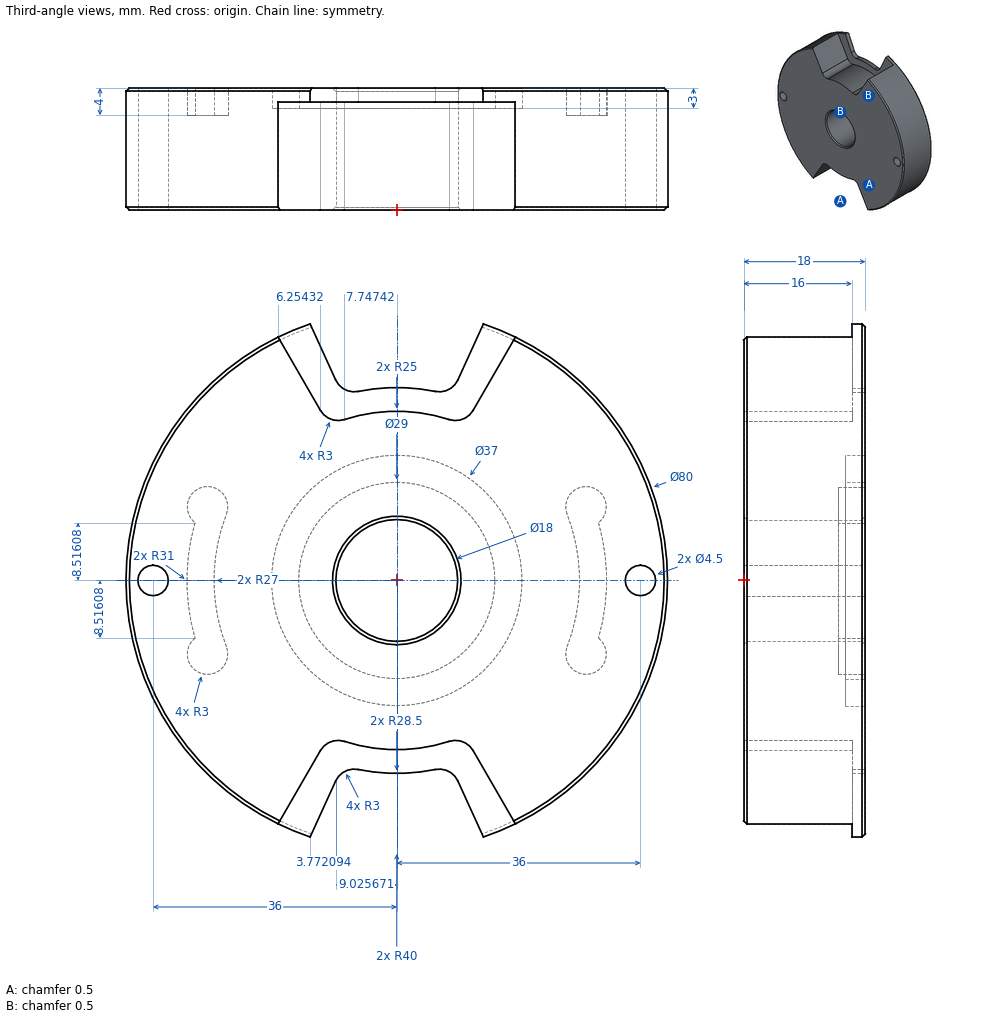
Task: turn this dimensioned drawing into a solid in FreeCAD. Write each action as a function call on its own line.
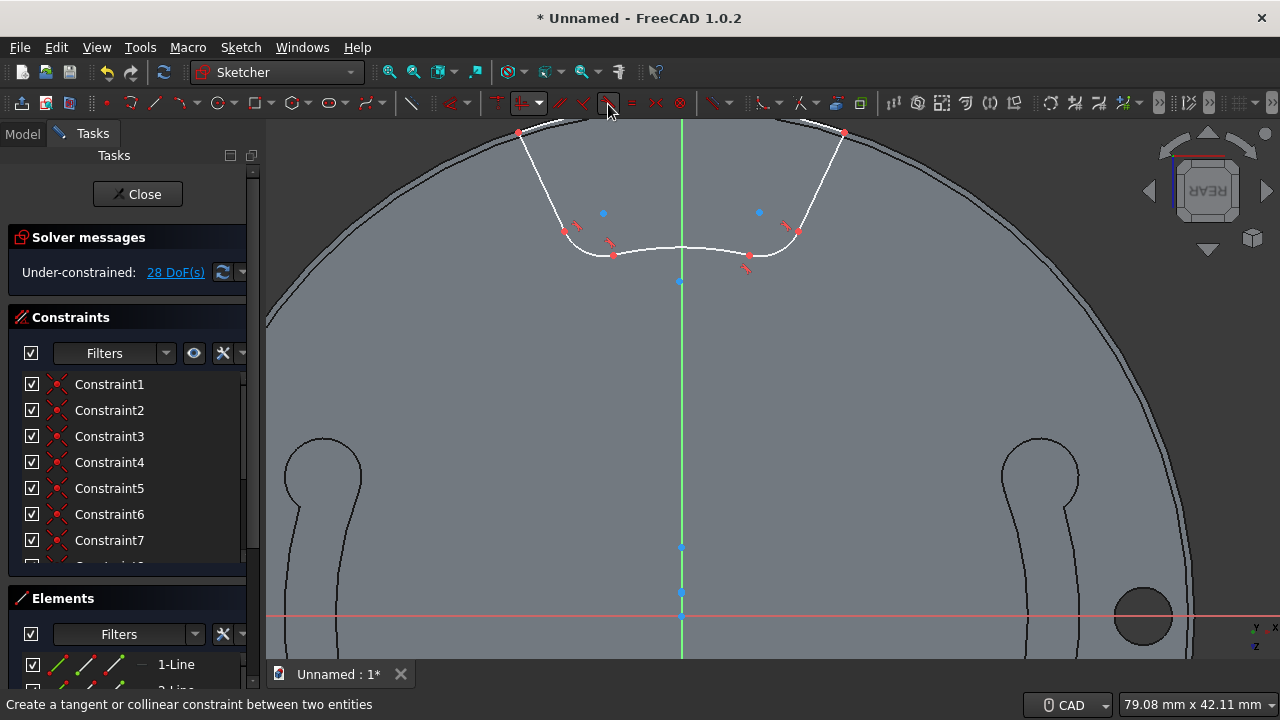
scroll(718, 257, down, 5)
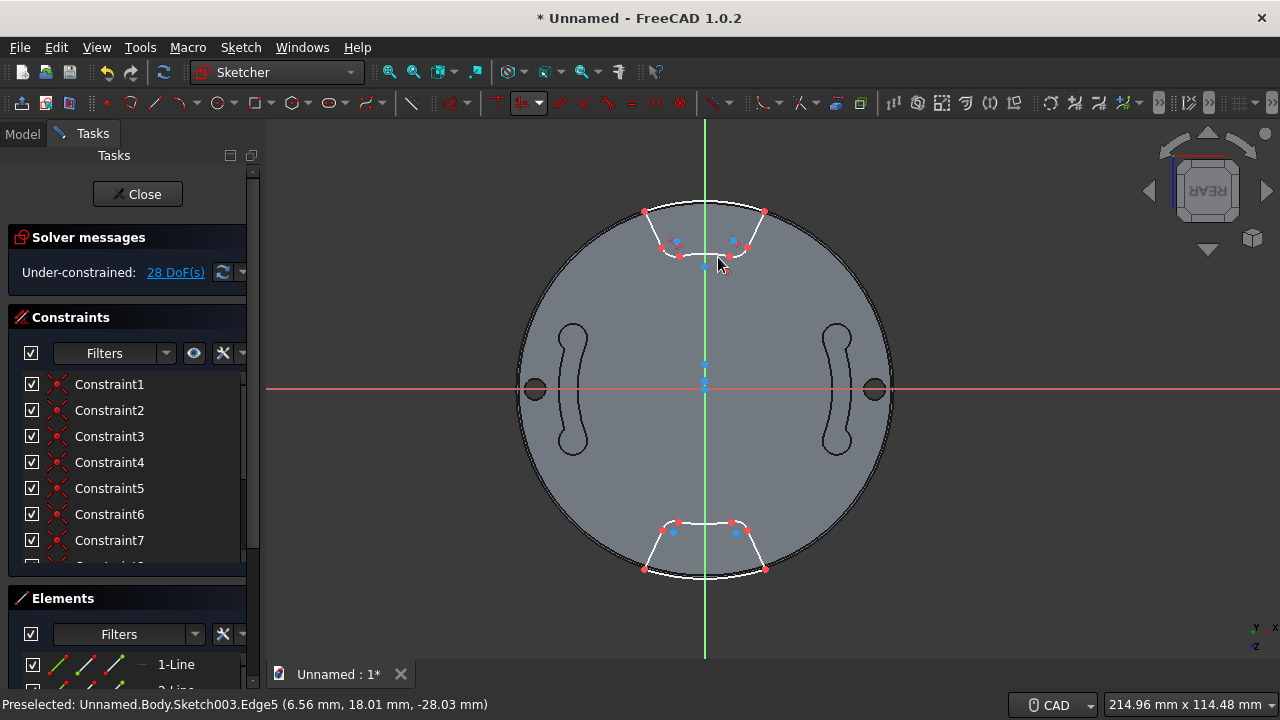
click(760, 558)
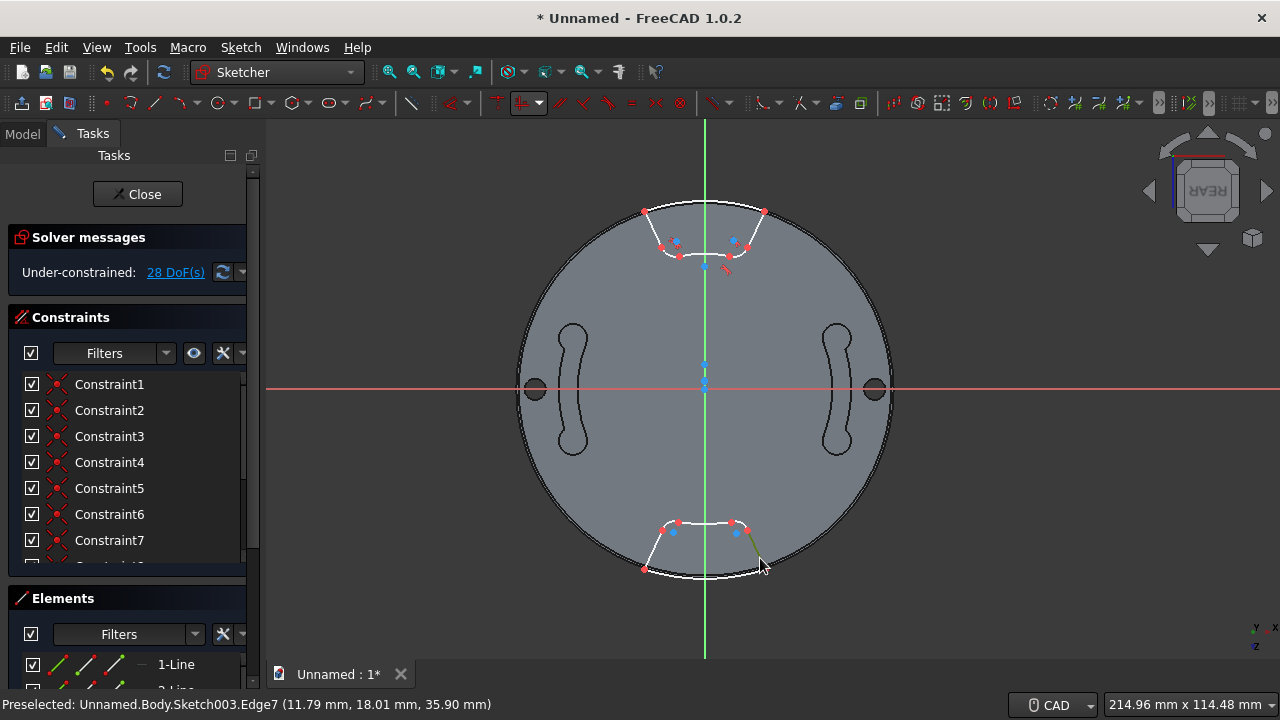
scroll(741, 523, up, 2)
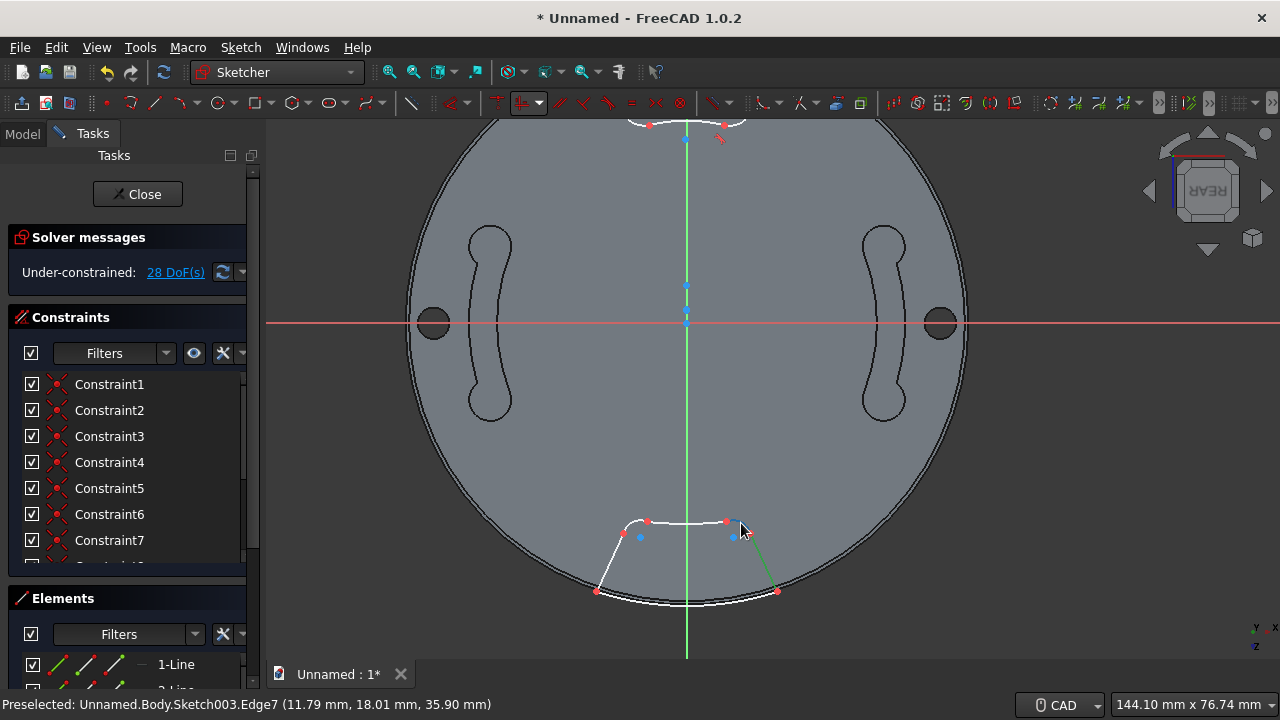
click(741, 522)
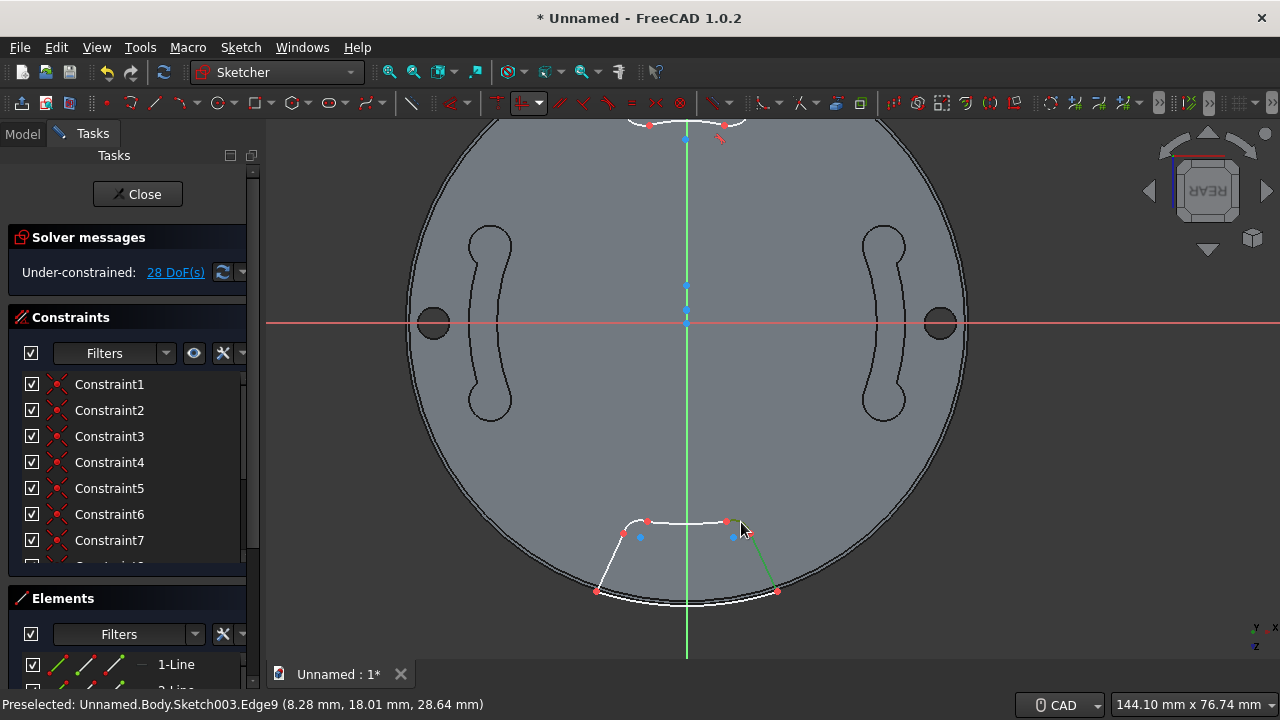
click(608, 104)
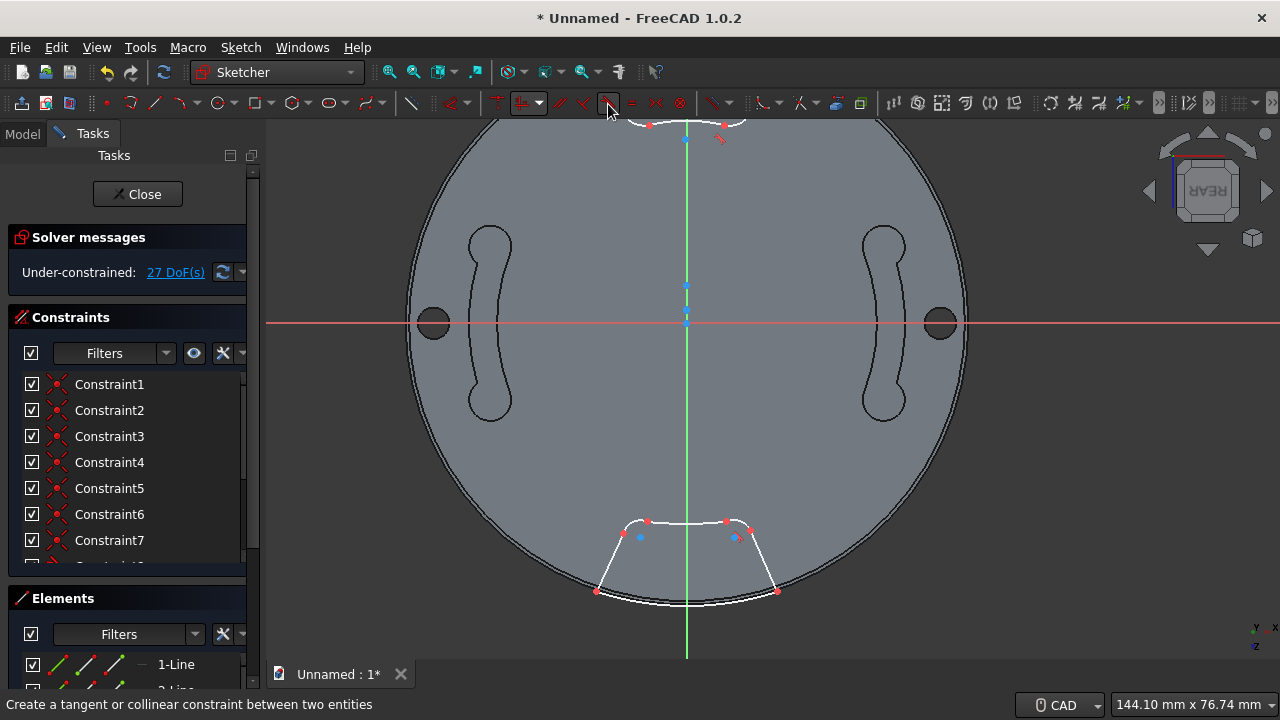
click(616, 551)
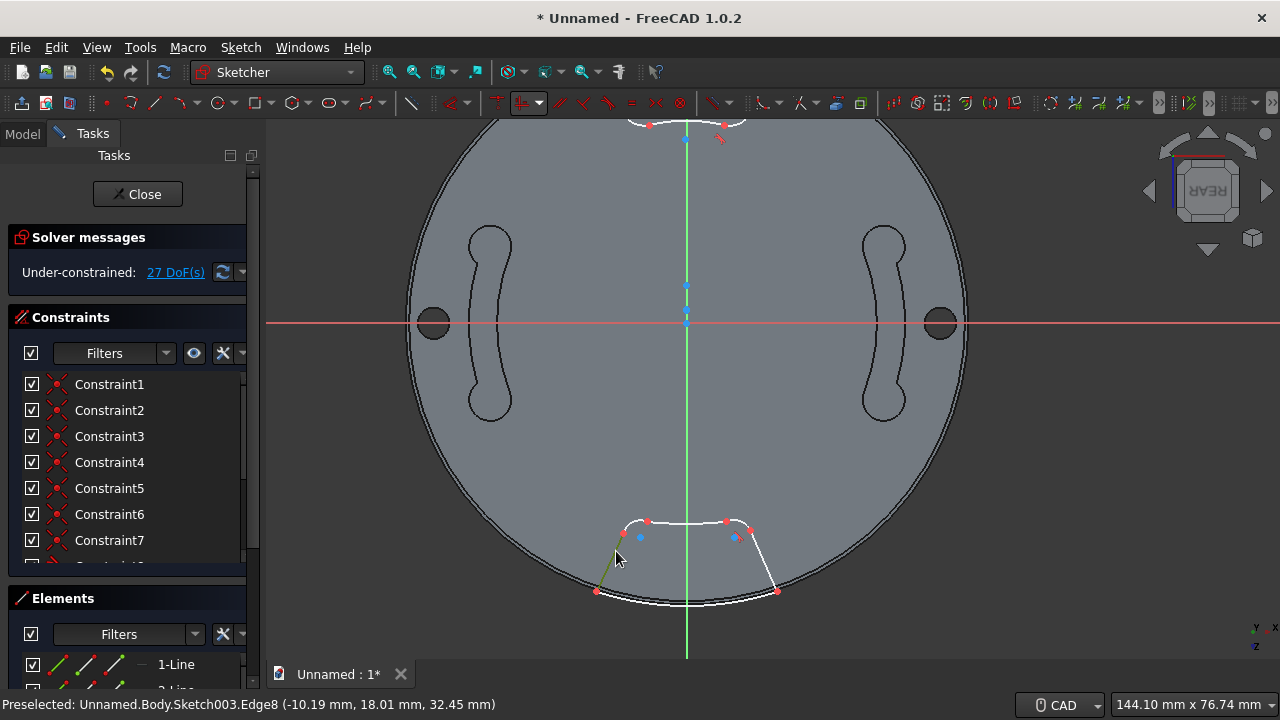
scroll(639, 520, up, 3)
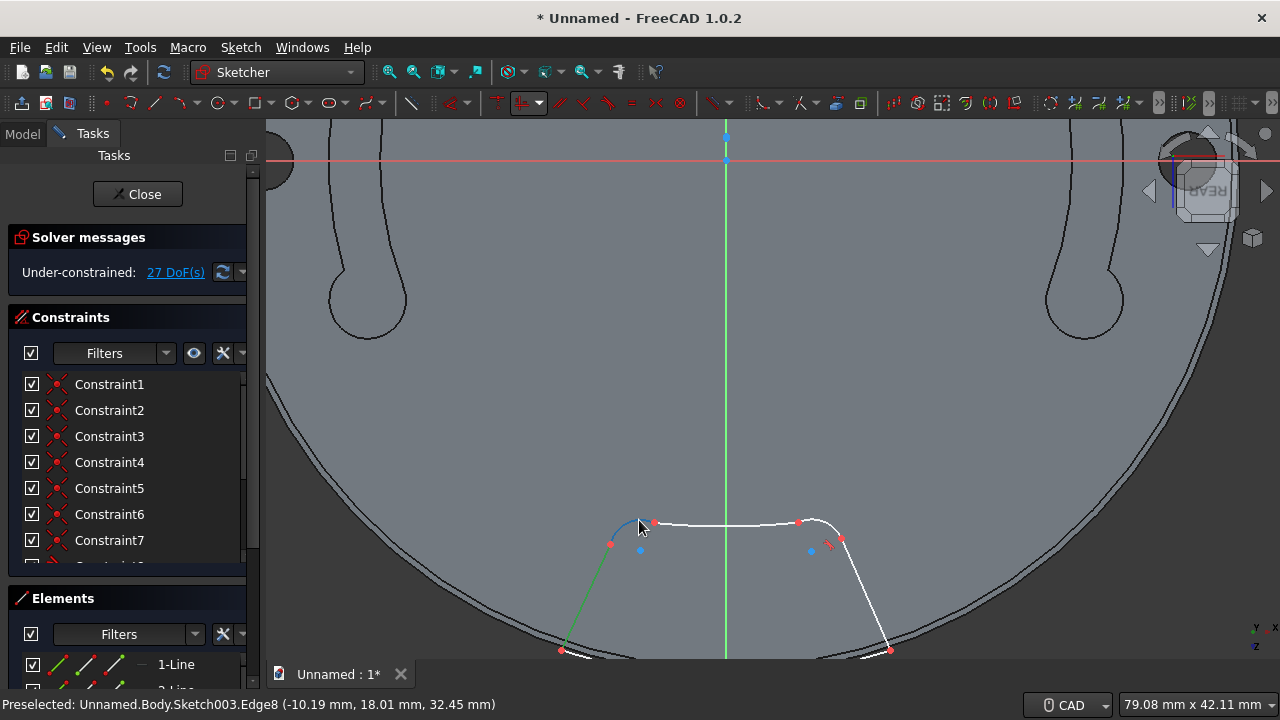
click(638, 520)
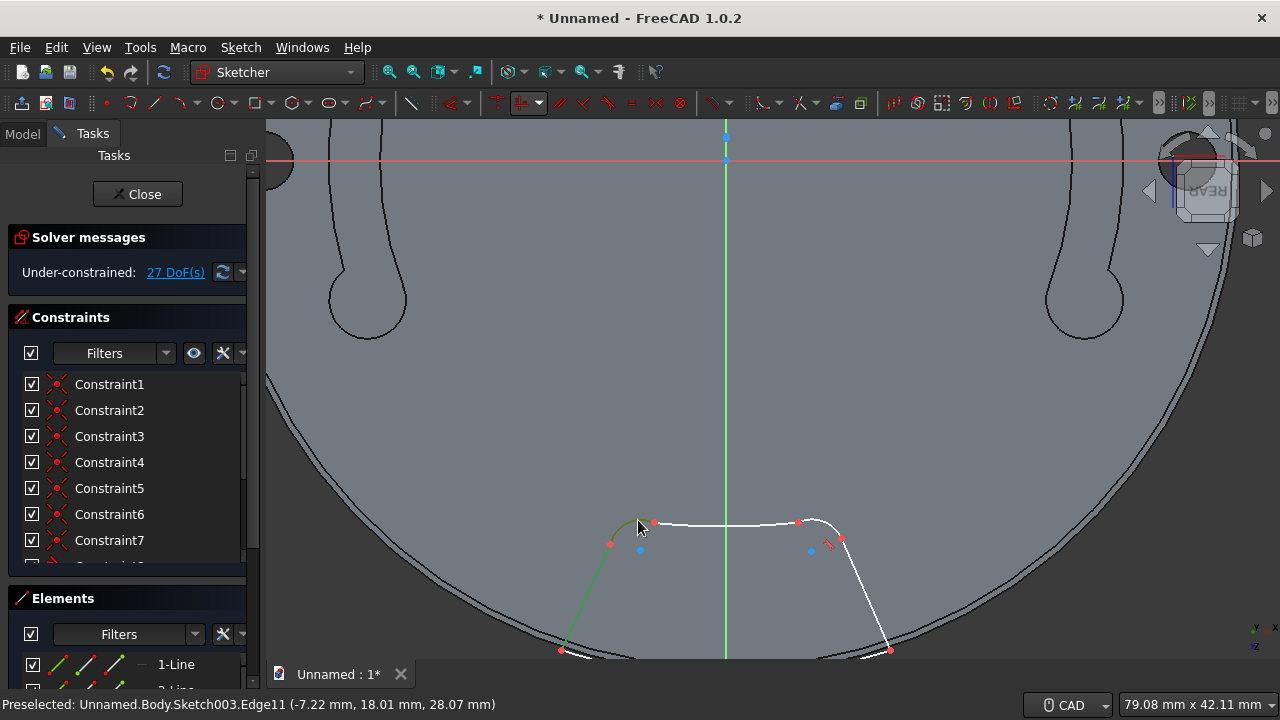
click(608, 104)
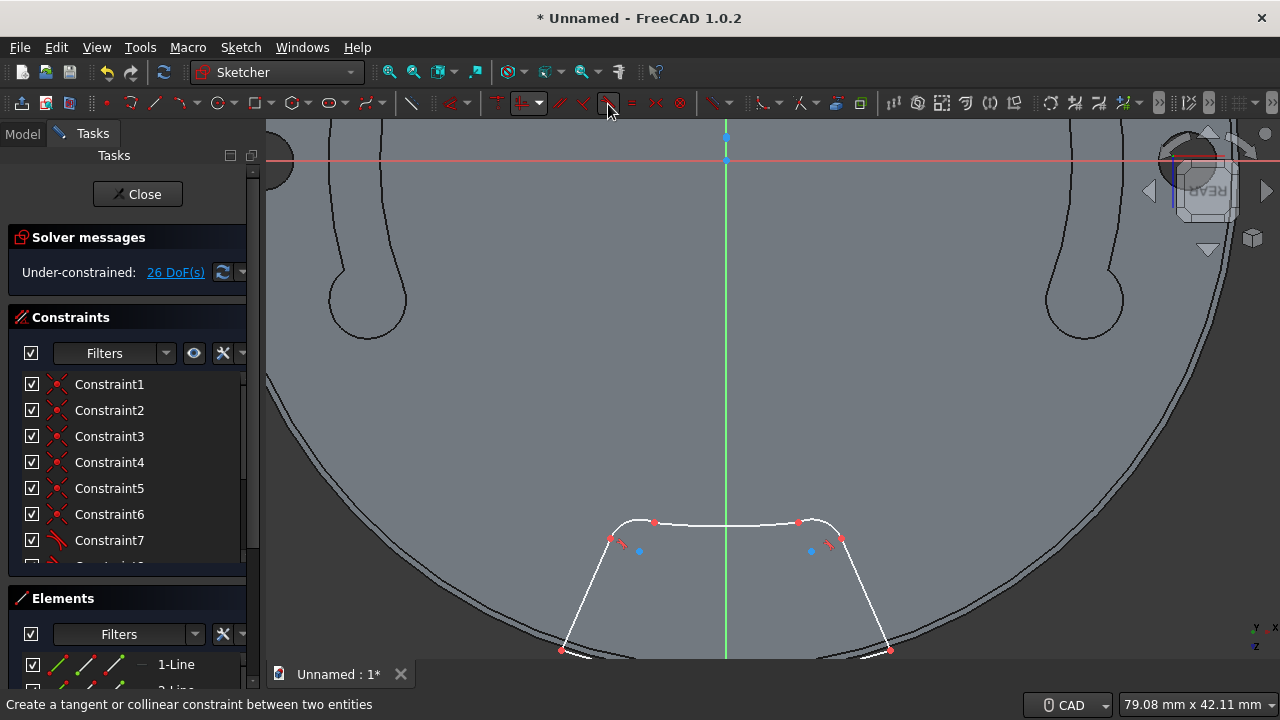
click(832, 527)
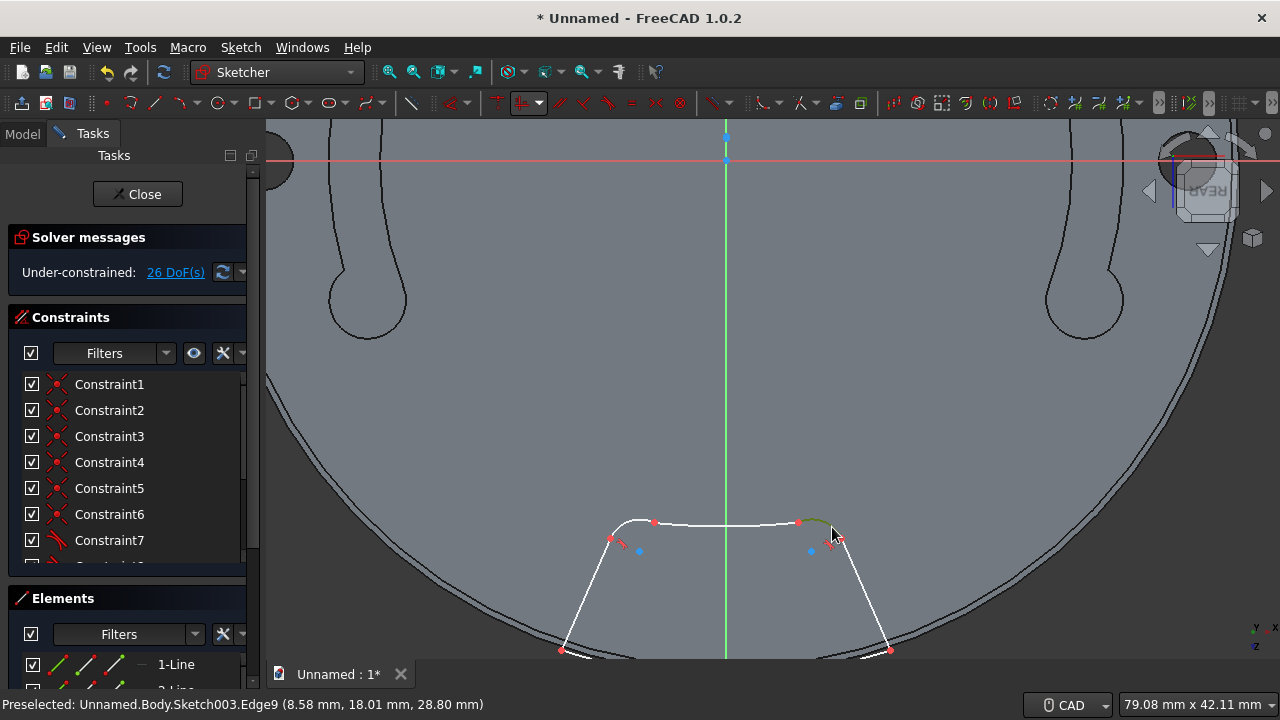
click(697, 526)